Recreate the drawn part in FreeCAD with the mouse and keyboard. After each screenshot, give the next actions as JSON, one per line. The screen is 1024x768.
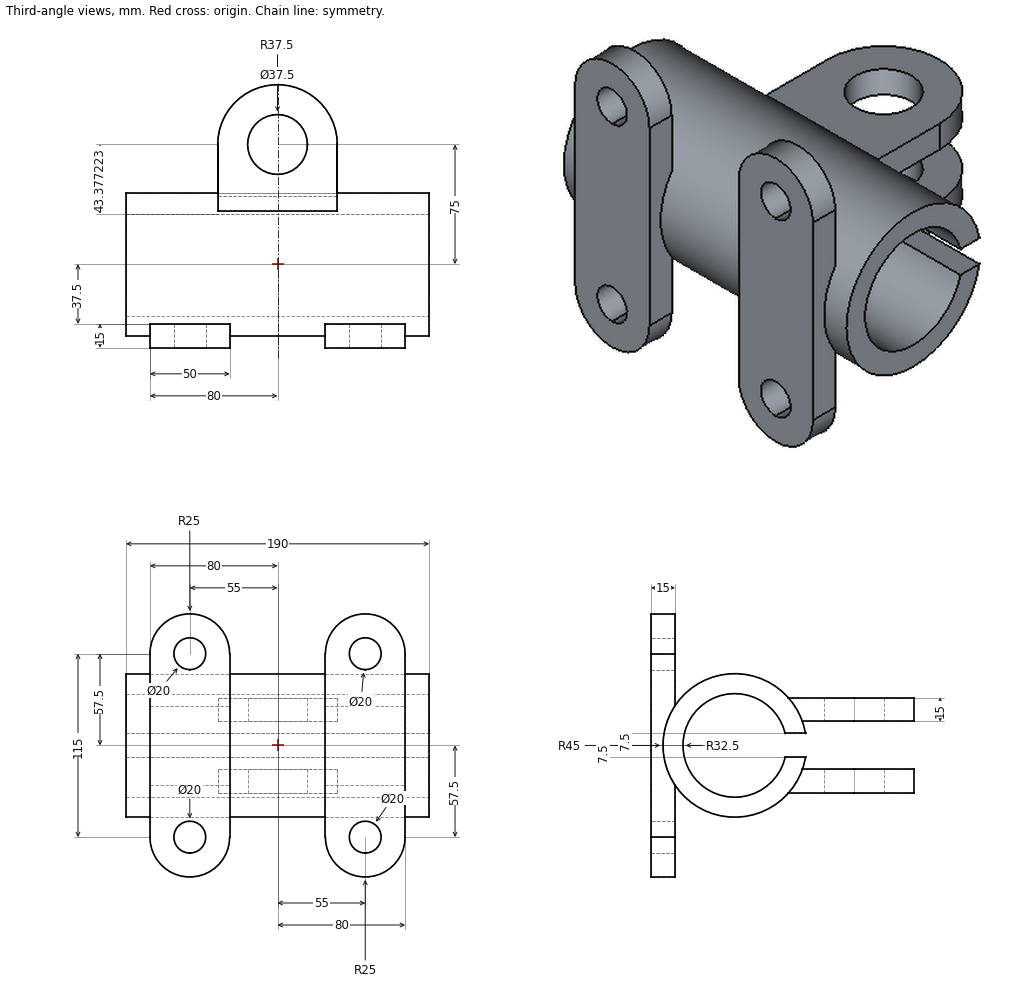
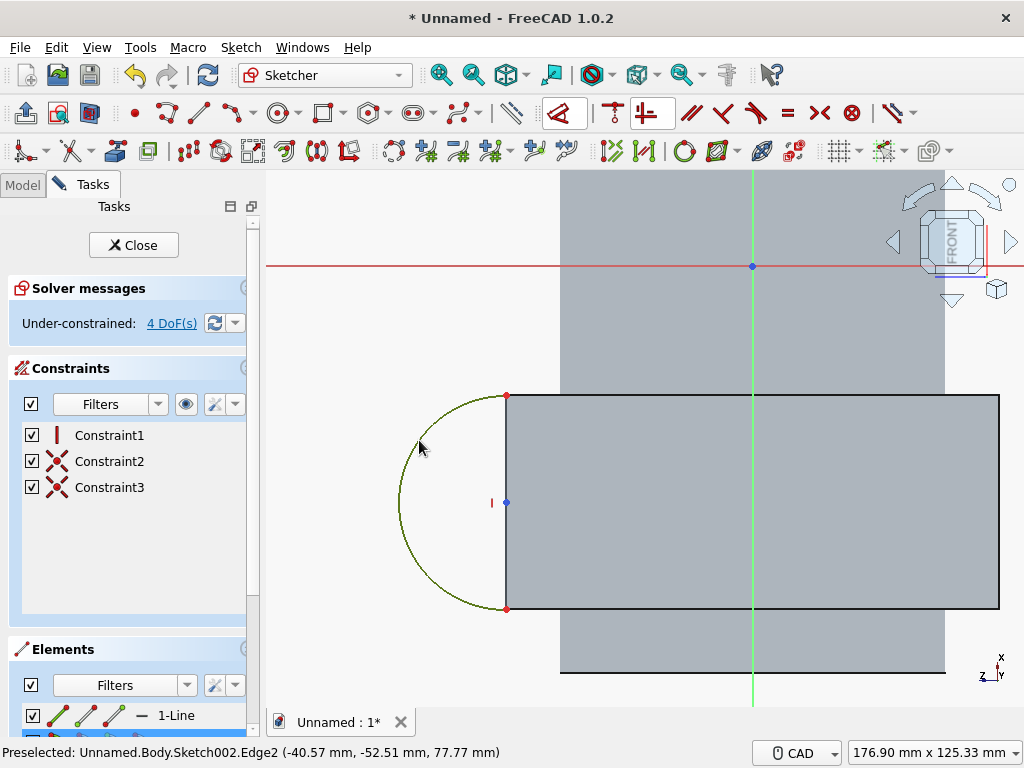
{"action": "left_click", "coordinate": [582, 114]}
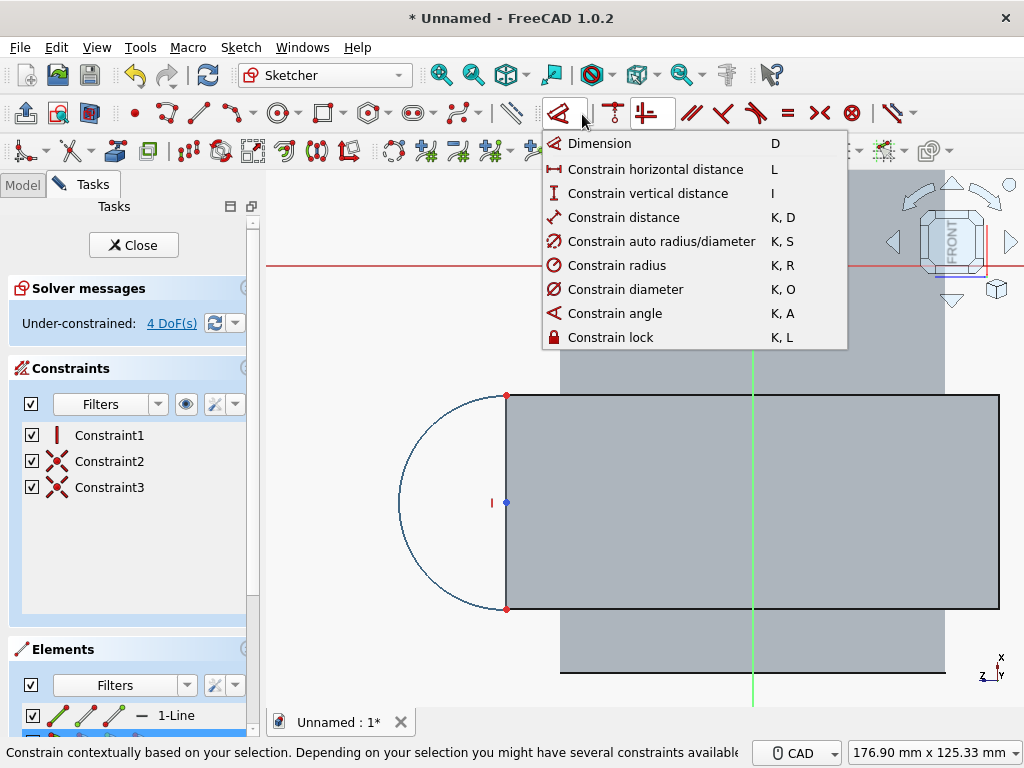
{"action": "left_click", "coordinate": [695, 265]}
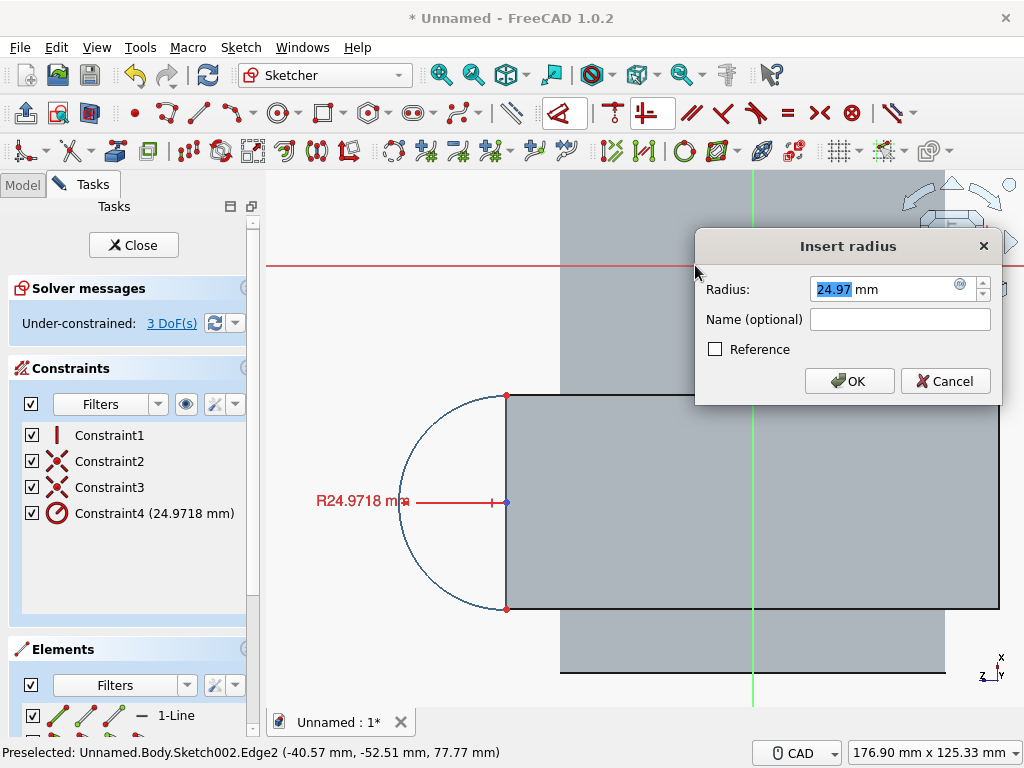
{"action": "type", "text": "25"}
{"action": "key", "text": "Return"}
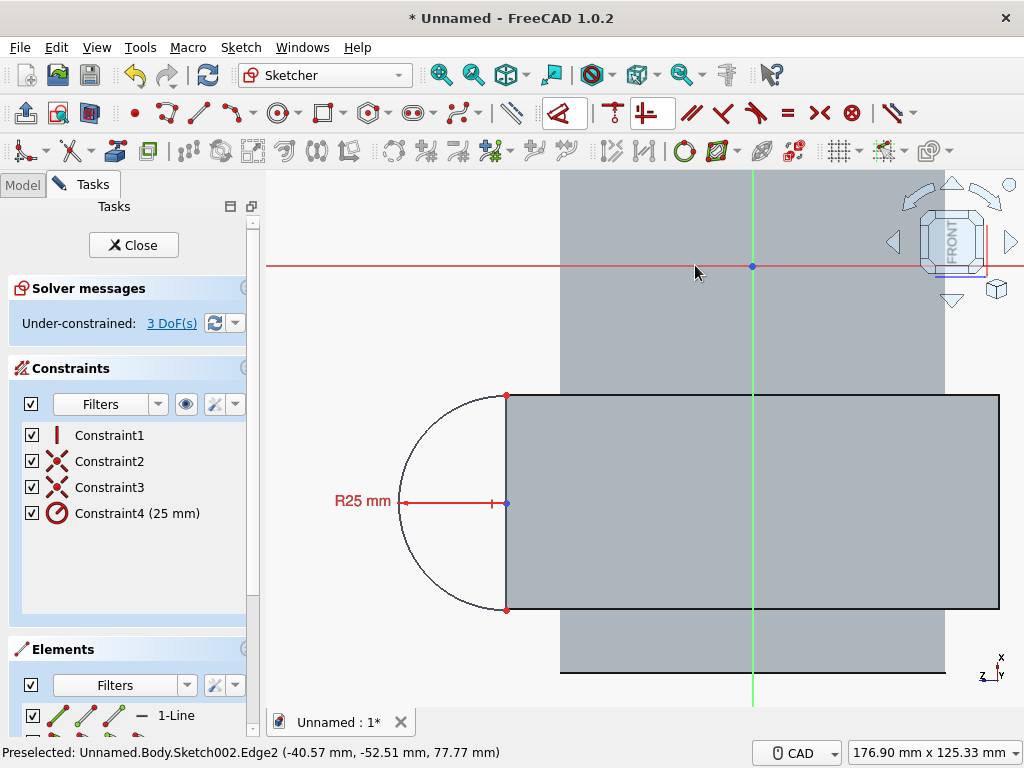
{"action": "left_click", "coordinate": [506, 610]}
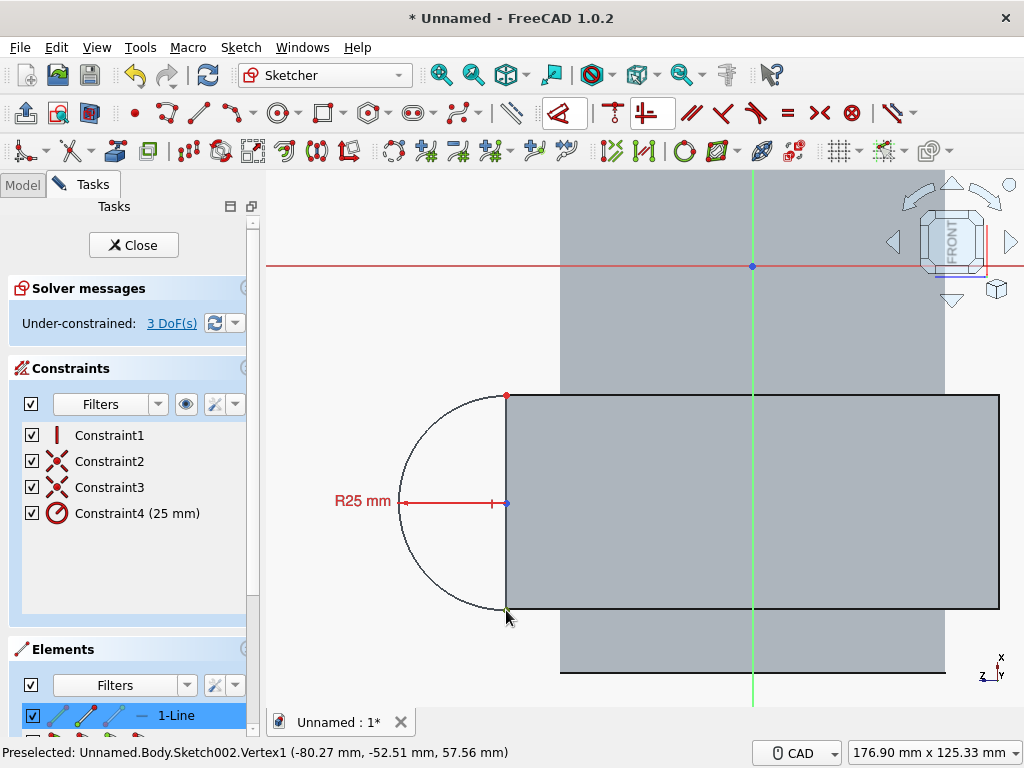
{"action": "key", "text": "i"}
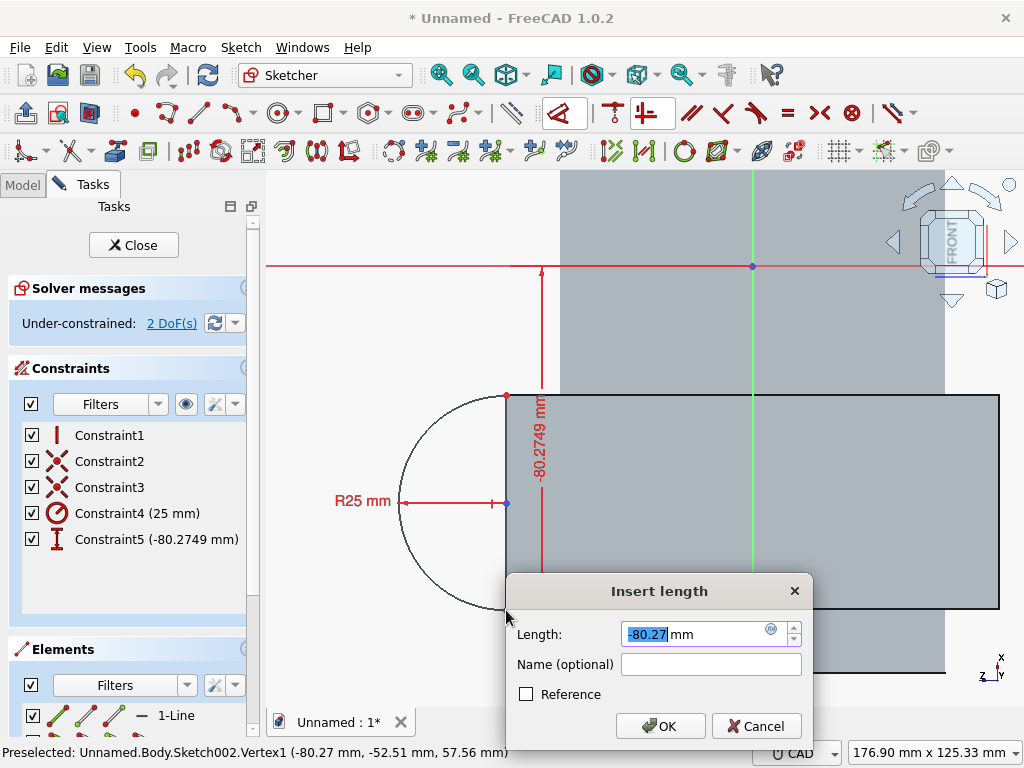
{"action": "type", "text": "-80"}
{"action": "key", "text": "Return"}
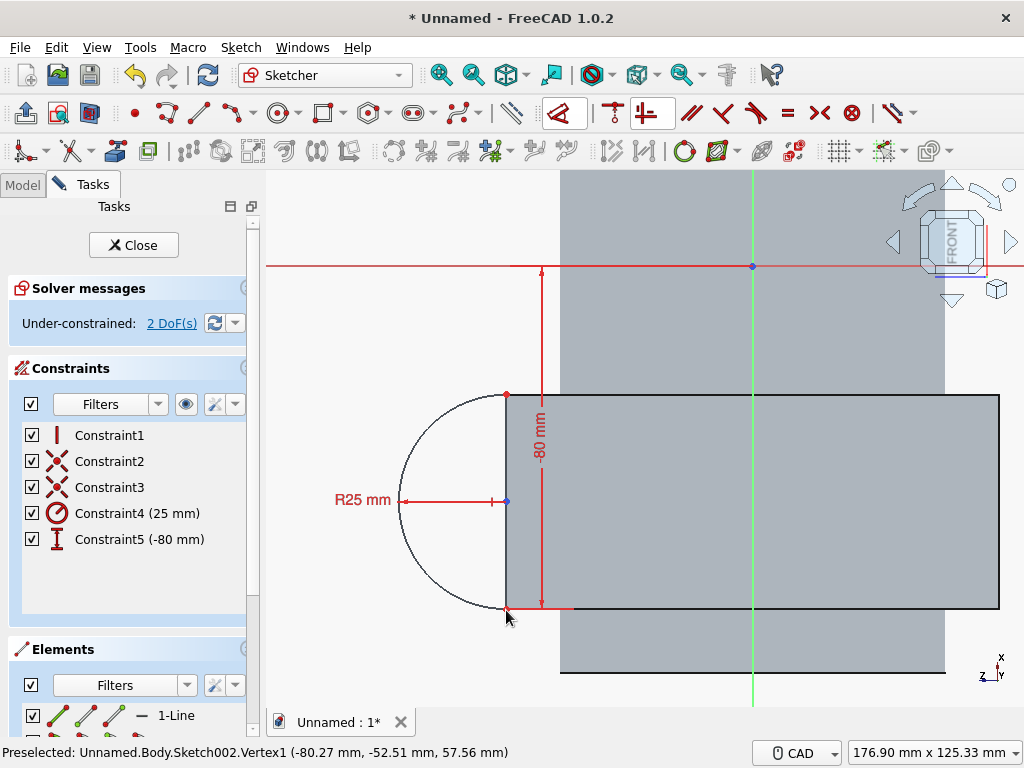
{"action": "left_click", "coordinate": [506, 609]}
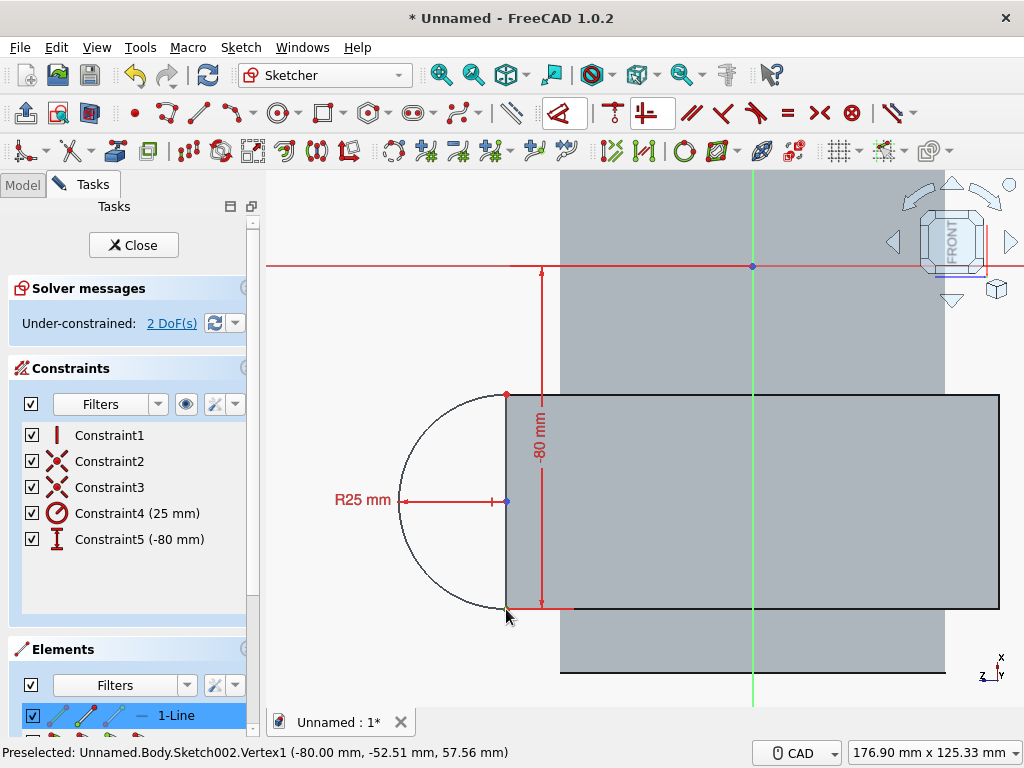
{"action": "left_click", "coordinate": [582, 114]}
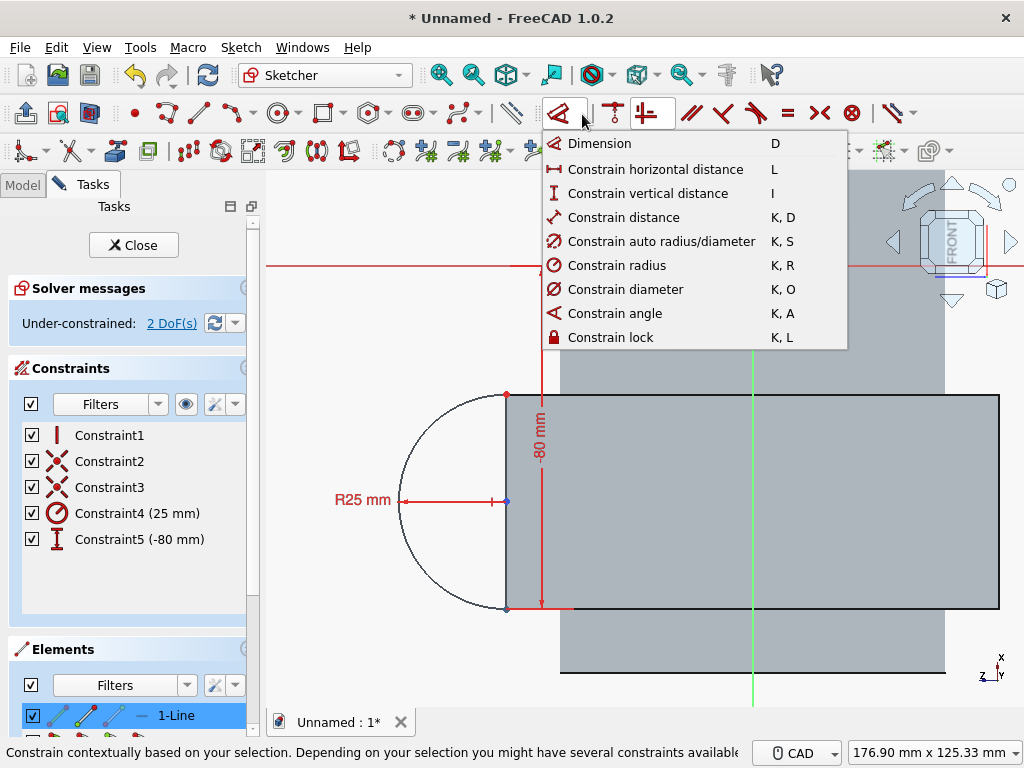
{"action": "left_click", "coordinate": [695, 169]}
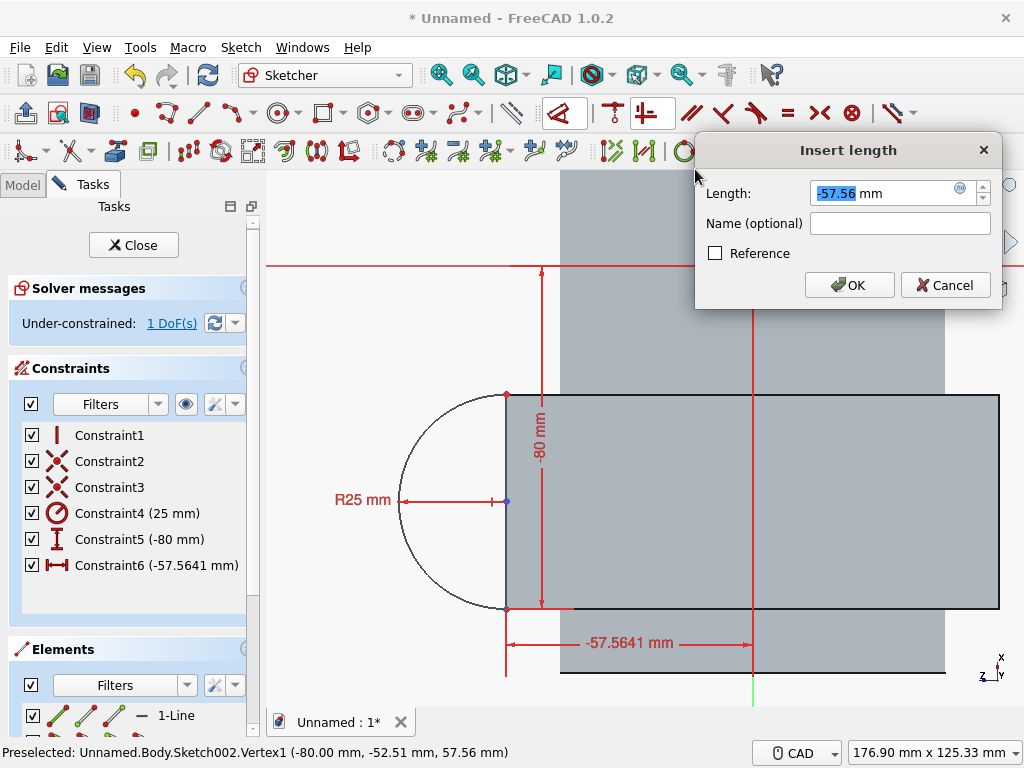
{"action": "type", "text": "-57.5"}
{"action": "key", "text": "Return"}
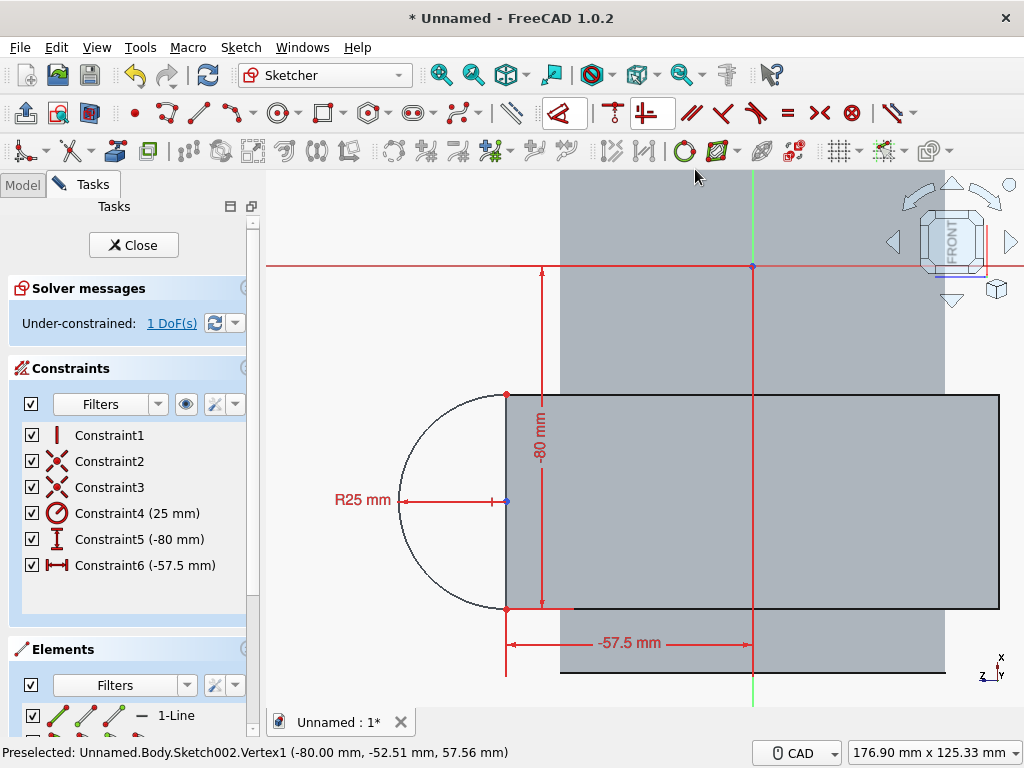
{"action": "left_click", "coordinate": [506, 502]}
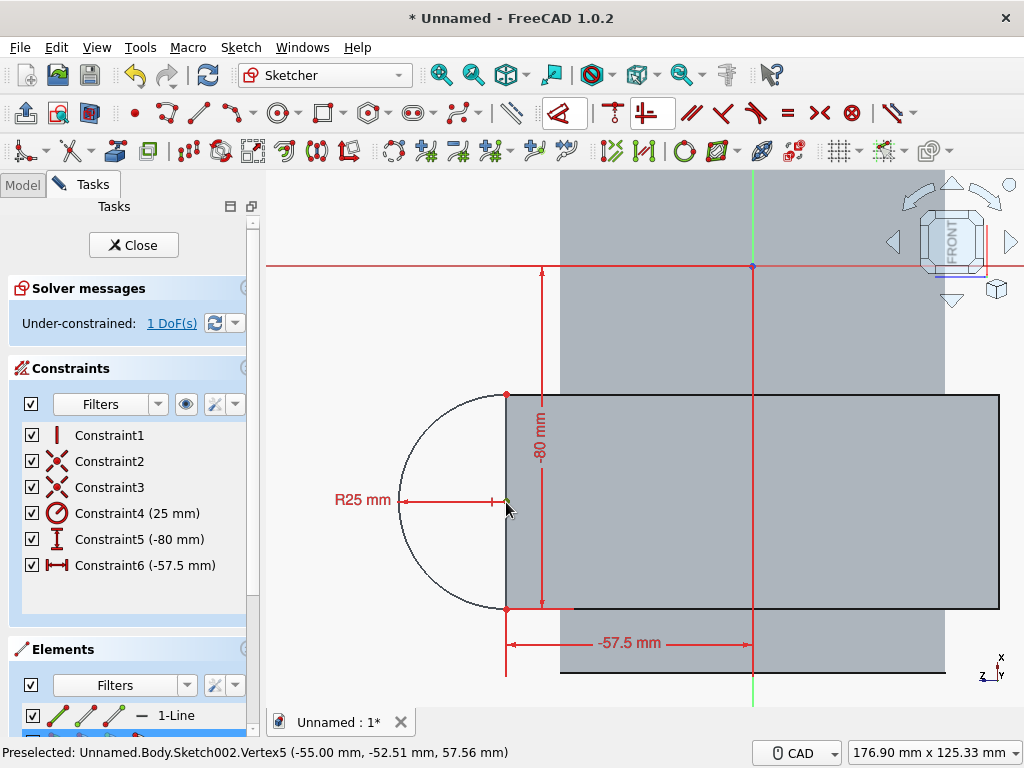
{"action": "key", "text": "l"}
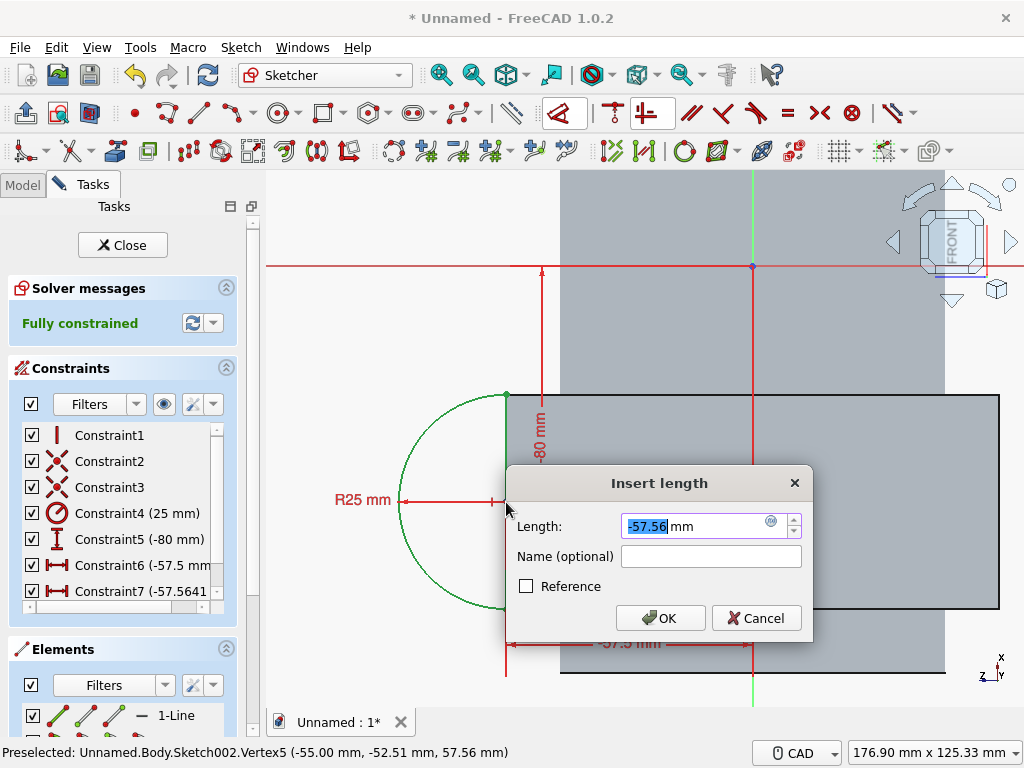
{"action": "type", "text": "-57.5"}
{"action": "key", "text": "Return"}